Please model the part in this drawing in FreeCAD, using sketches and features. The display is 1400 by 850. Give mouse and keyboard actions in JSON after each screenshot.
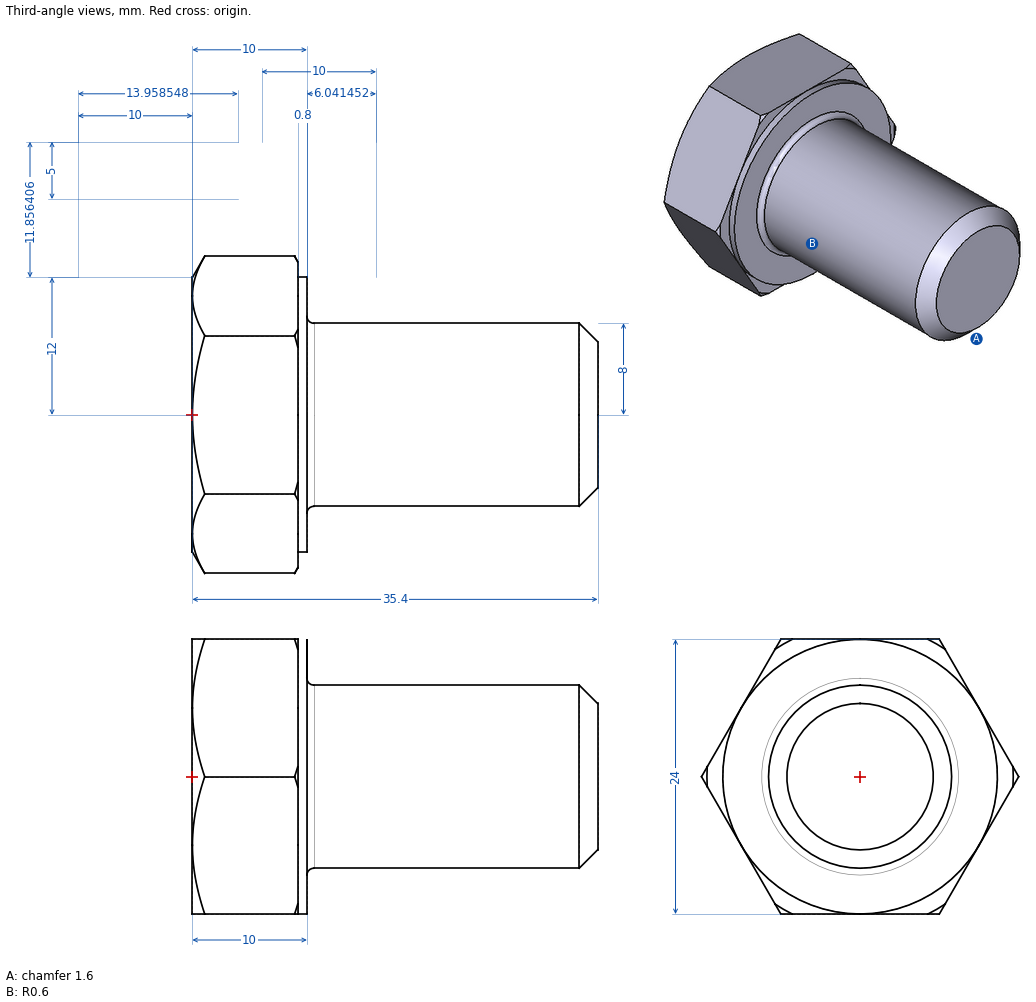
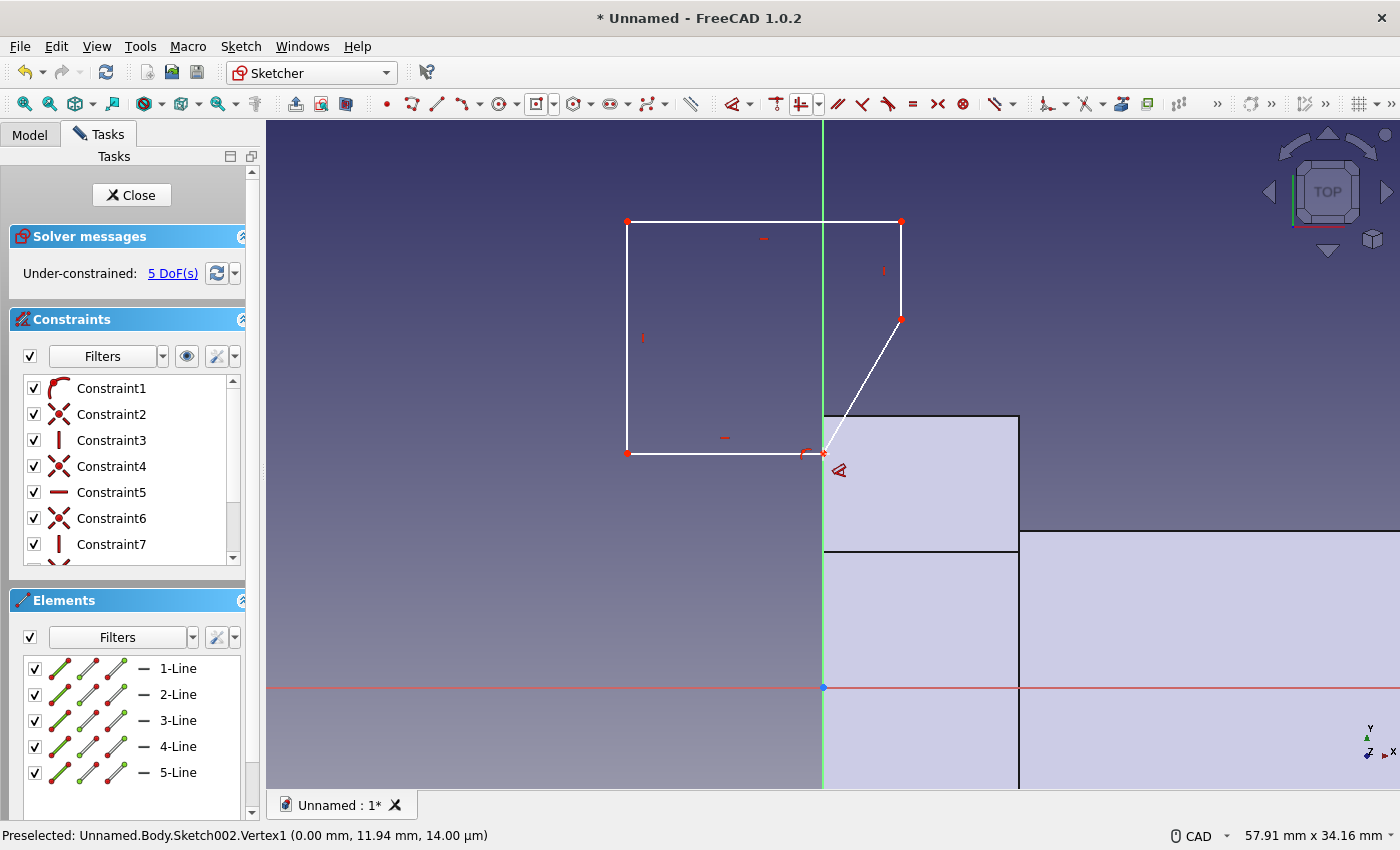
{"action": "left_click", "coordinate": [901, 291]}
{"action": "left_click", "coordinate": [935, 271]}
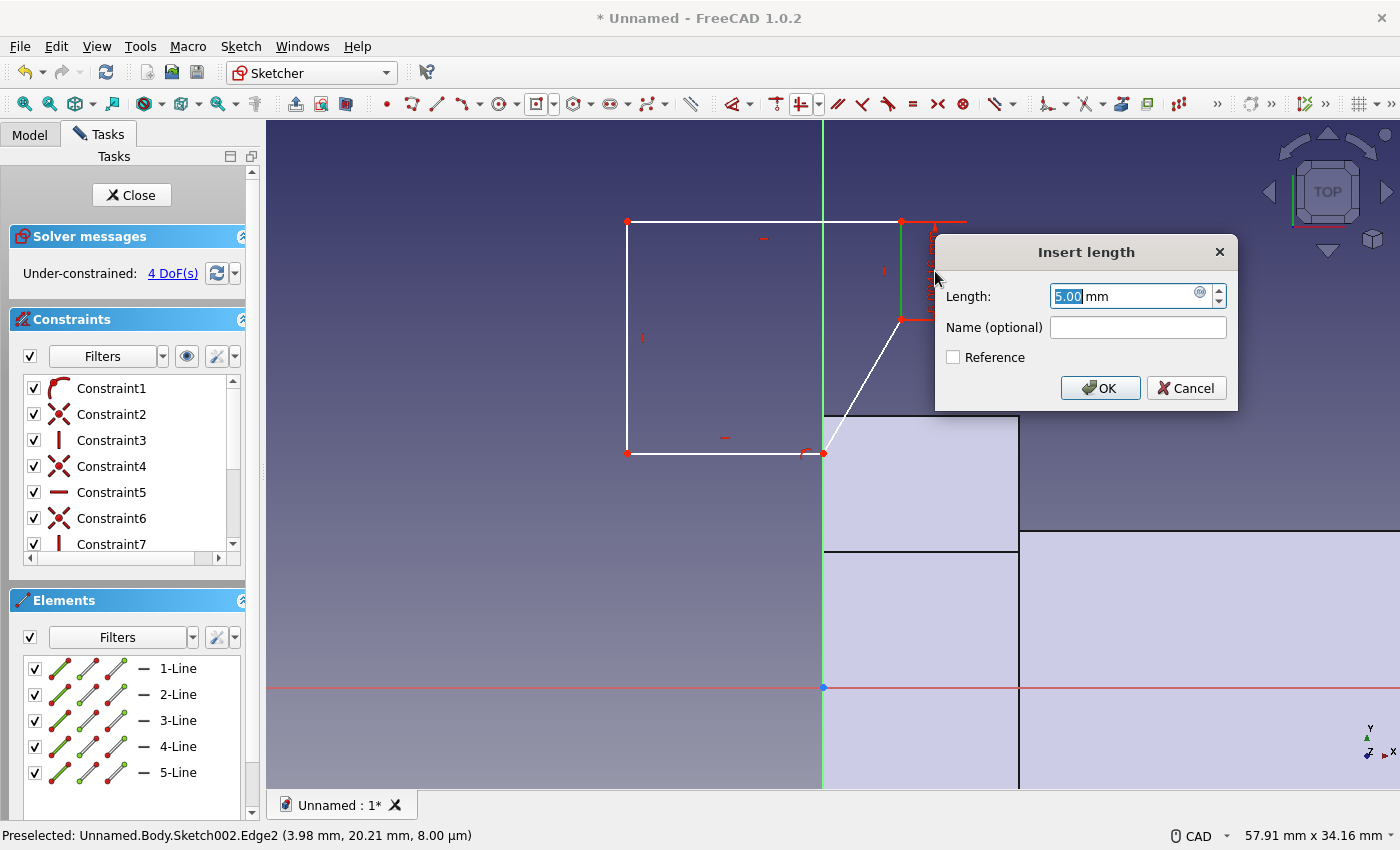
{"action": "type", "text": "5"}
{"action": "key", "text": "Return"}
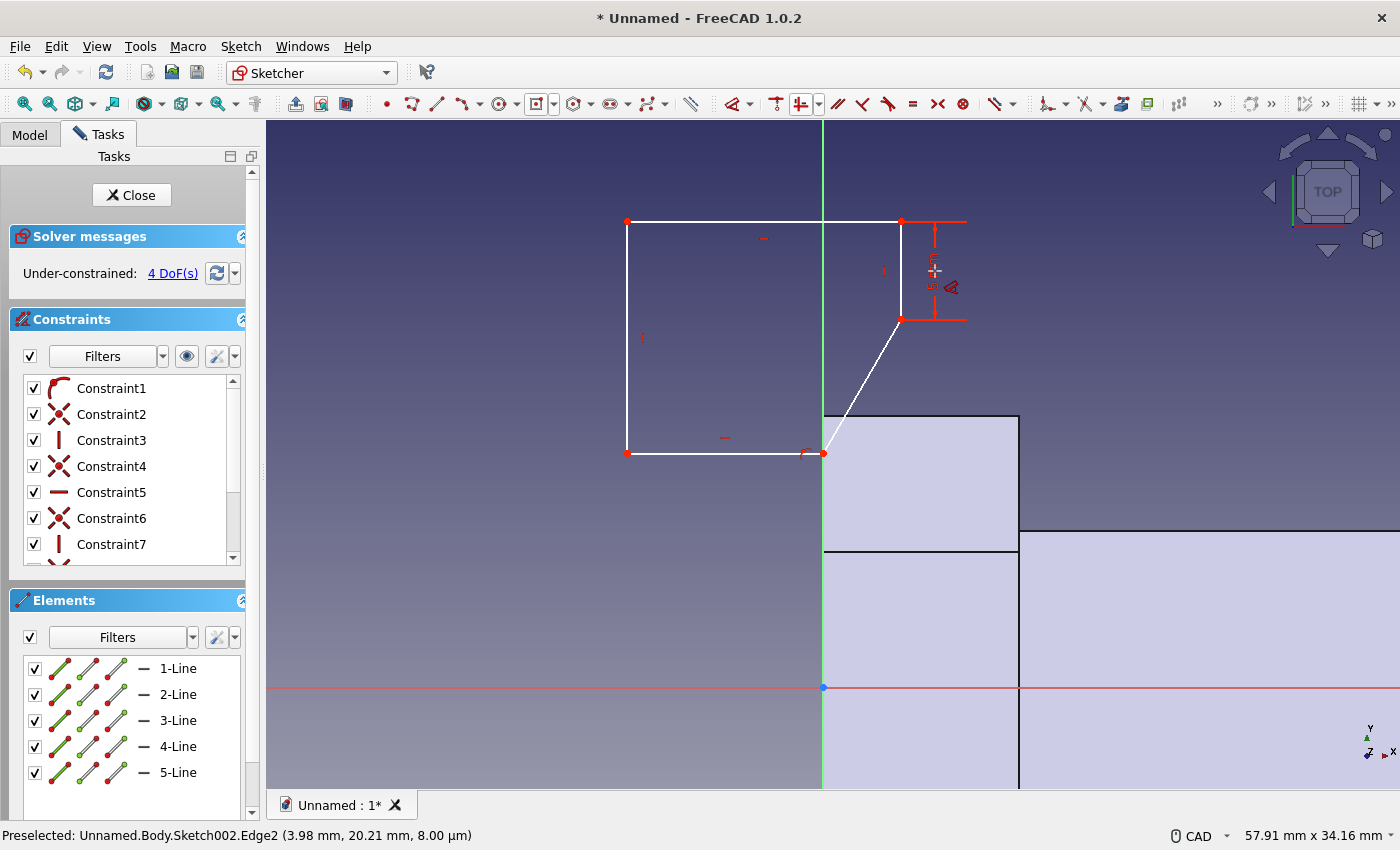
{"action": "left_click", "coordinate": [686, 454]}
{"action": "left_click", "coordinate": [725, 420]}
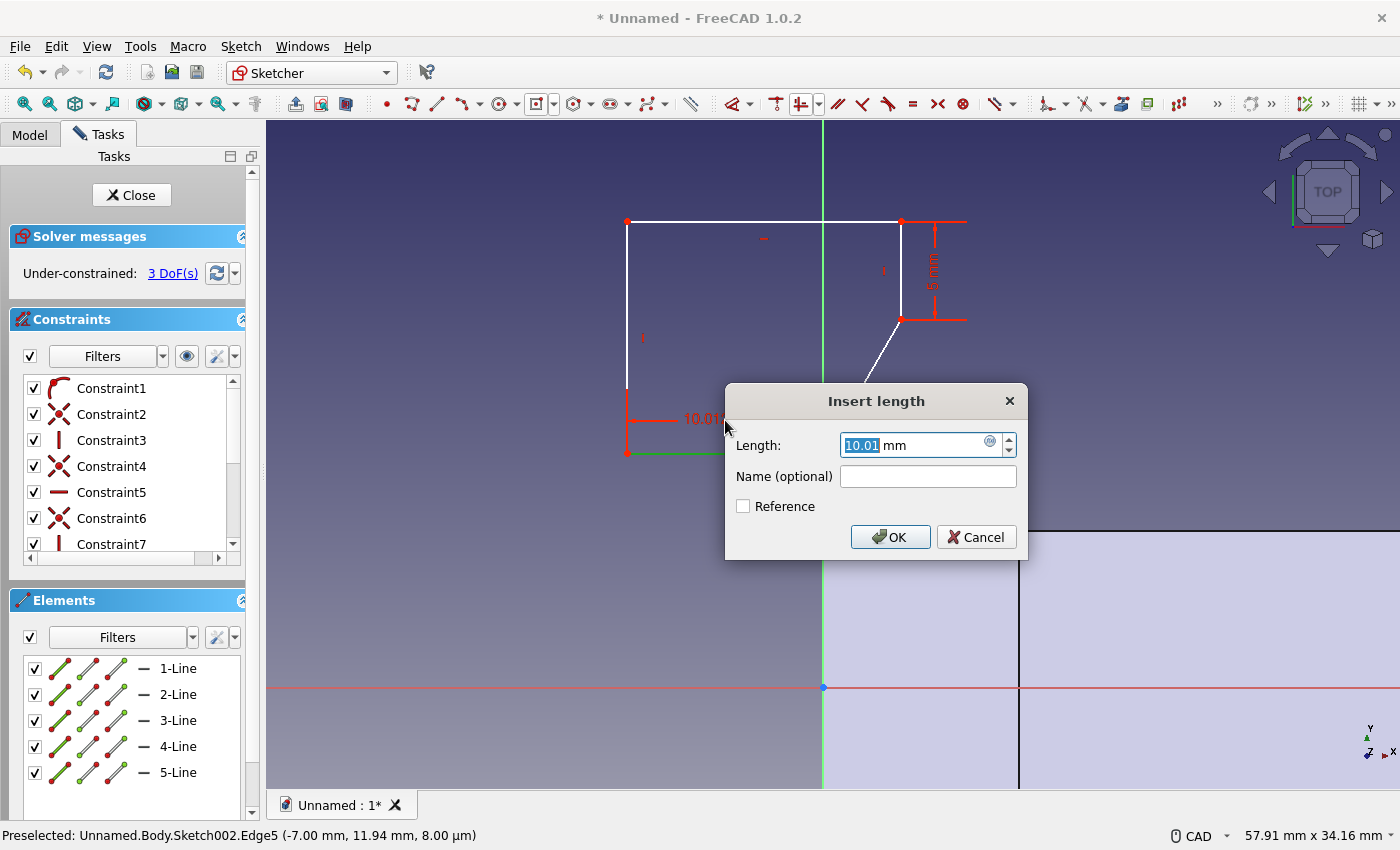
{"action": "type", "text": "10"}
{"action": "key", "text": "Return"}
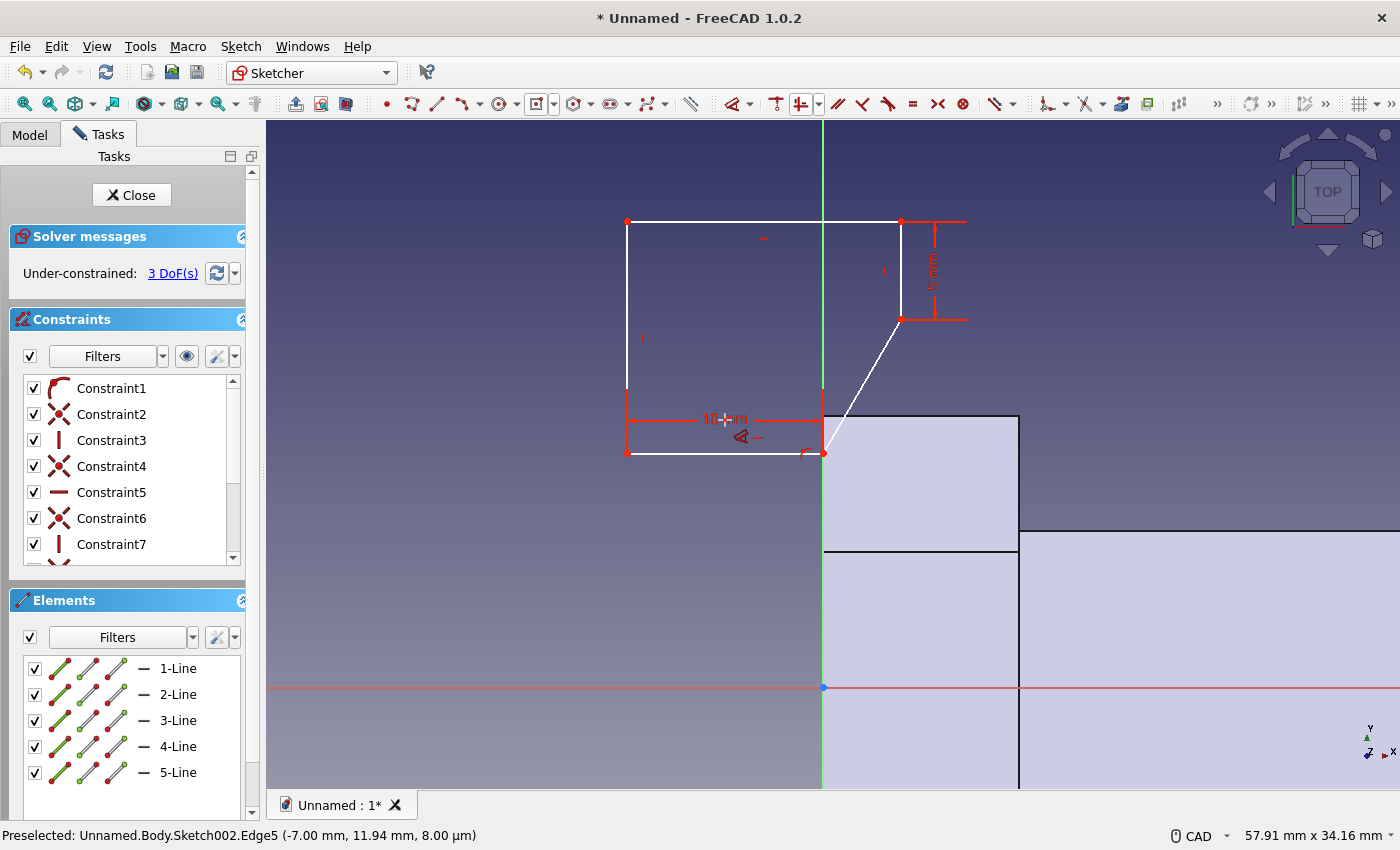
{"action": "left_click", "coordinate": [823, 454]}
{"action": "left_click", "coordinate": [857, 571]}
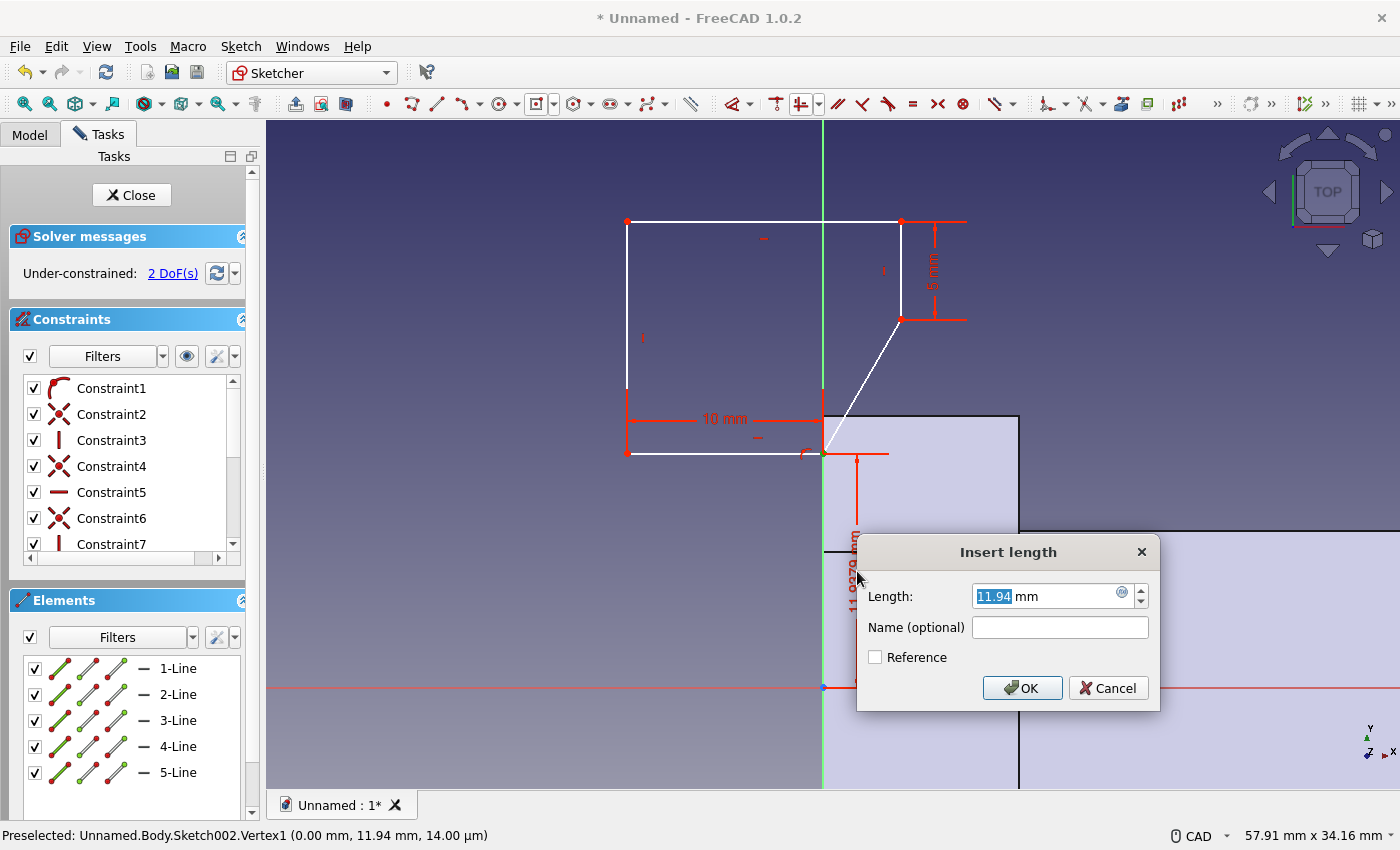
{"action": "type", "text": "12"}
{"action": "key", "text": "Return"}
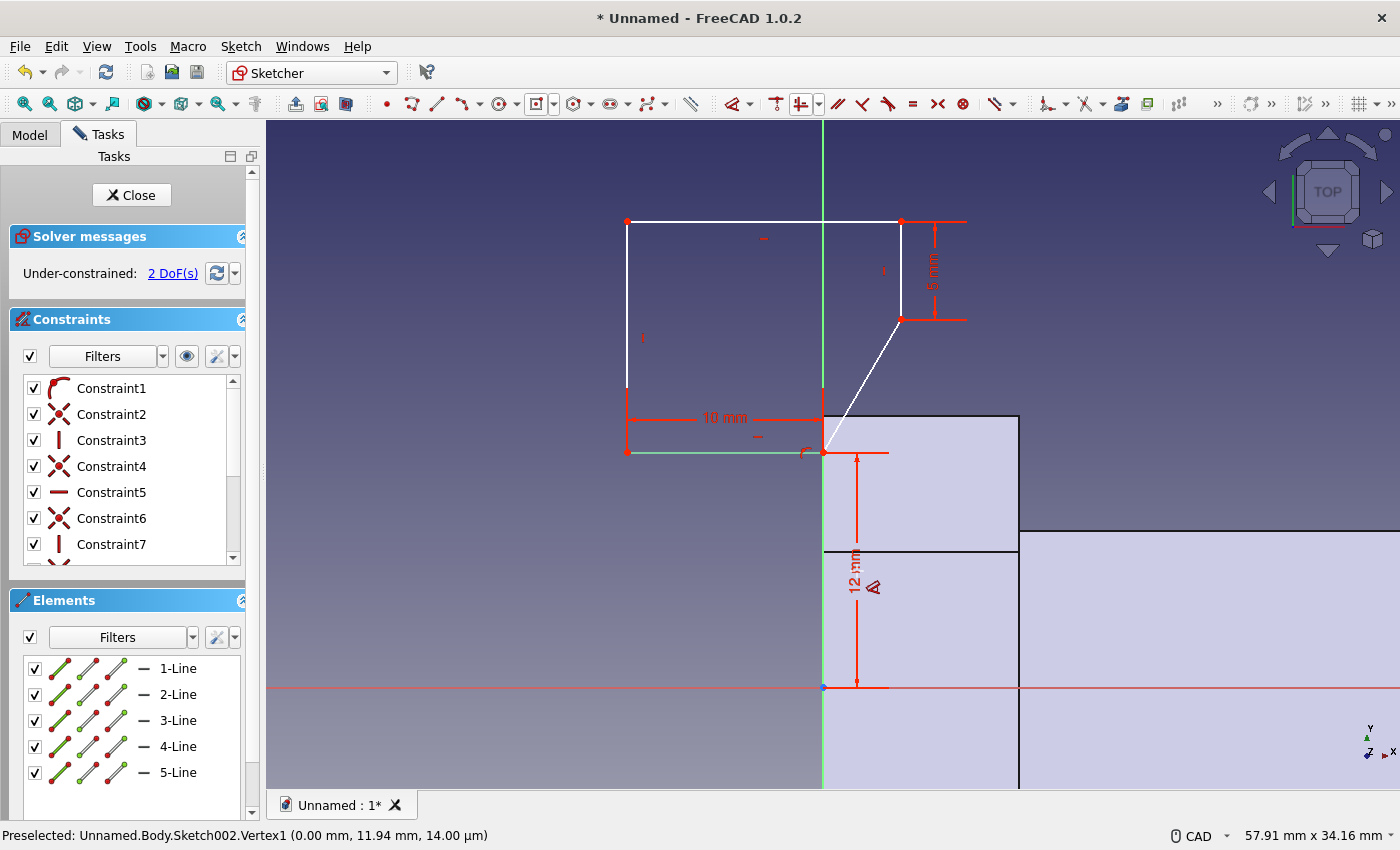
{"action": "left_click", "coordinate": [709, 222]}
{"action": "left_click", "coordinate": [764, 188]}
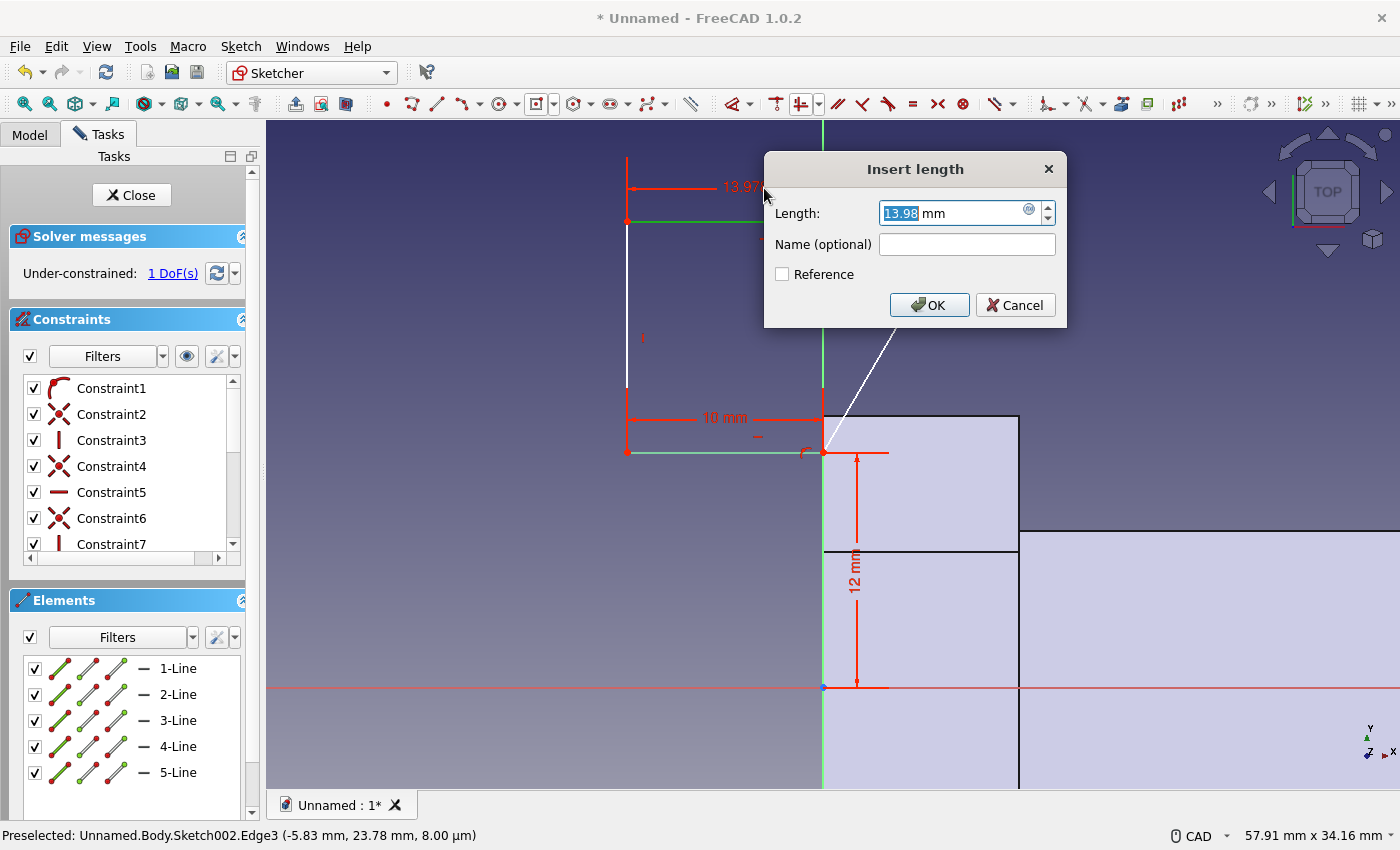
{"action": "type", "text": "13.958548"}
{"action": "key", "text": "Return"}